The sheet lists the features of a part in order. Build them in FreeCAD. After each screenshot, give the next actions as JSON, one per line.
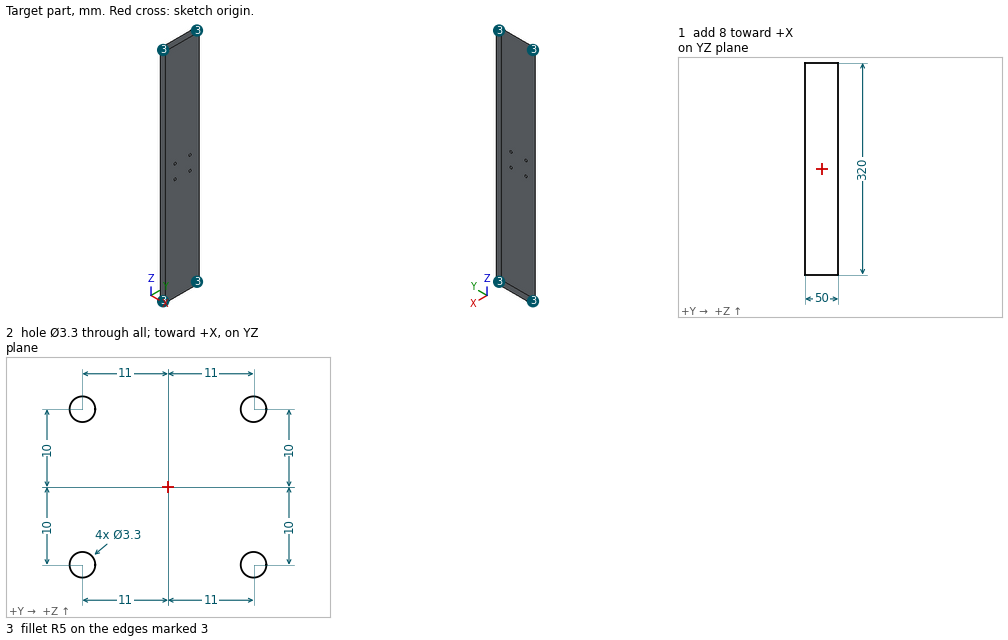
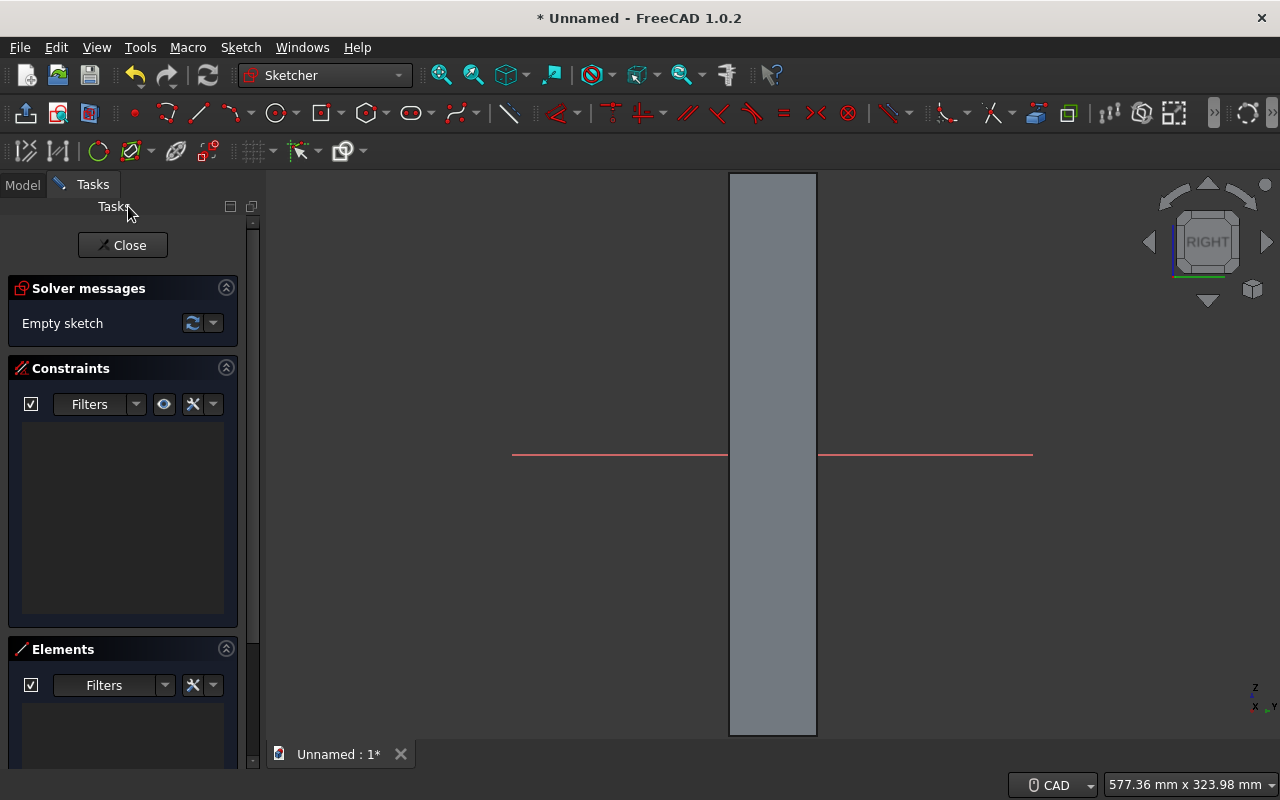
{"action": "left_click", "coordinate": [90, 114]}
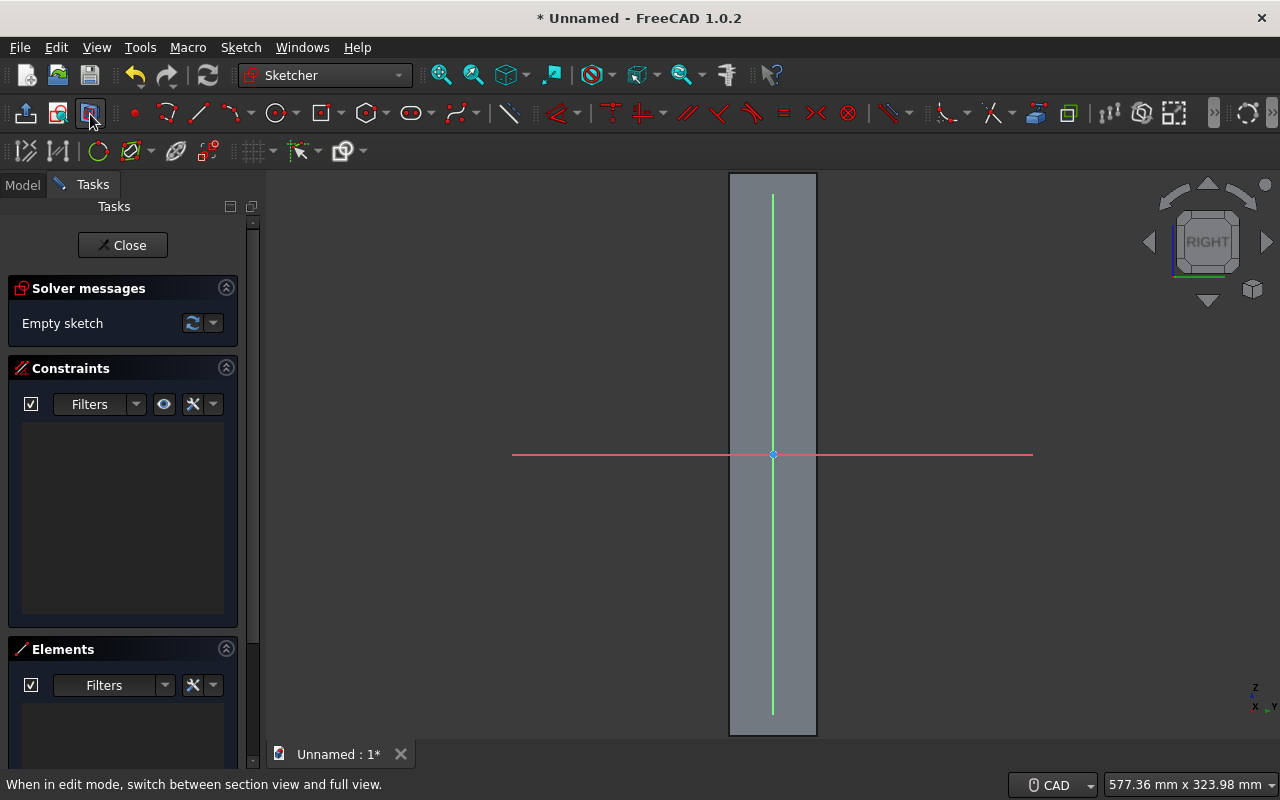
{"action": "scroll", "coordinate": [782, 454], "scroll_direction": "up", "scroll_amount": 11}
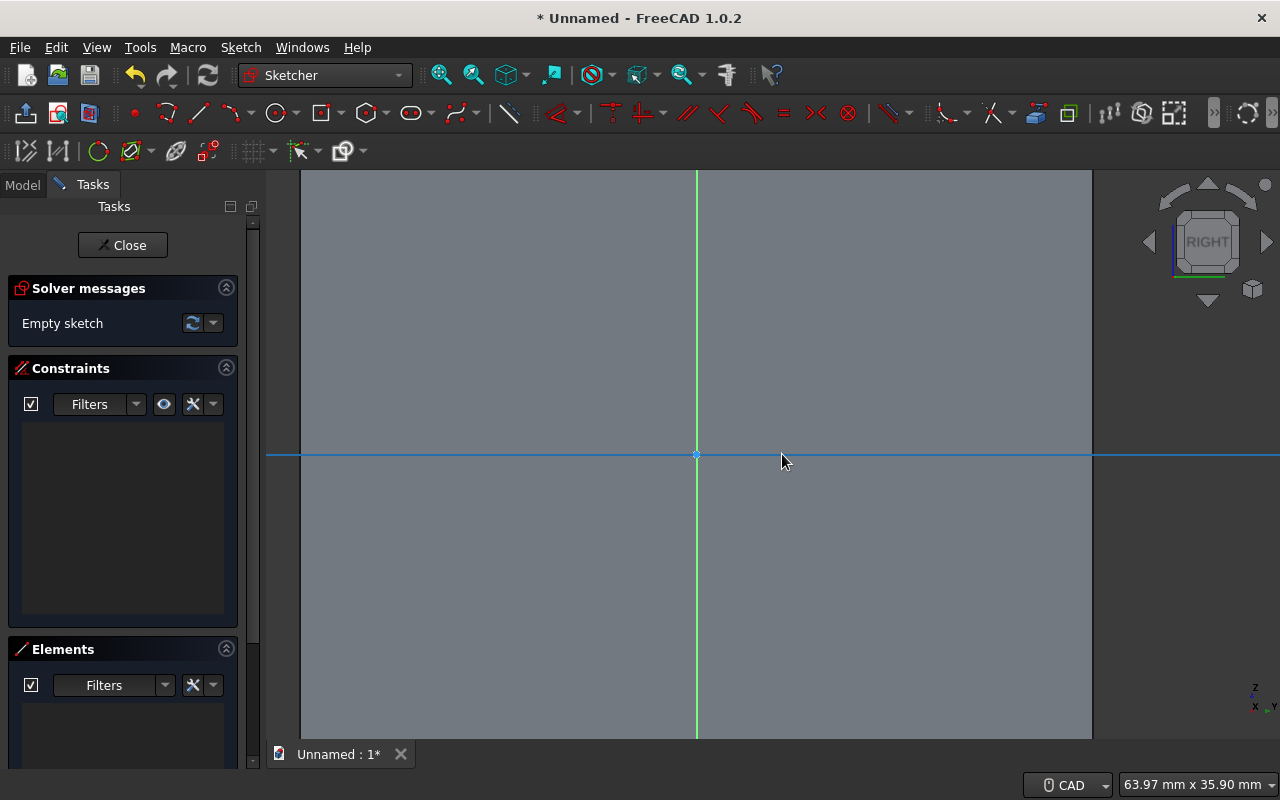
{"action": "left_click", "coordinate": [276, 114]}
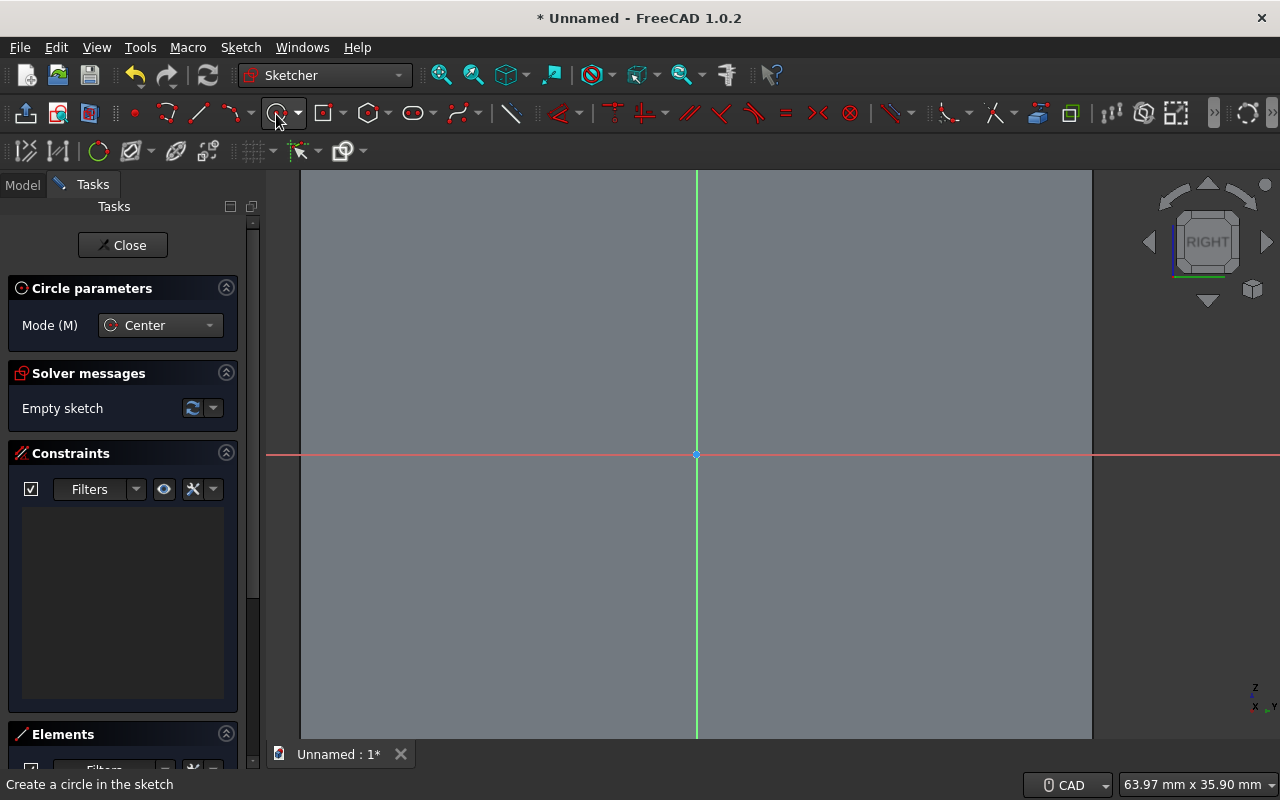
{"action": "left_click", "coordinate": [522, 613]}
{"action": "left_click", "coordinate": [541, 595]}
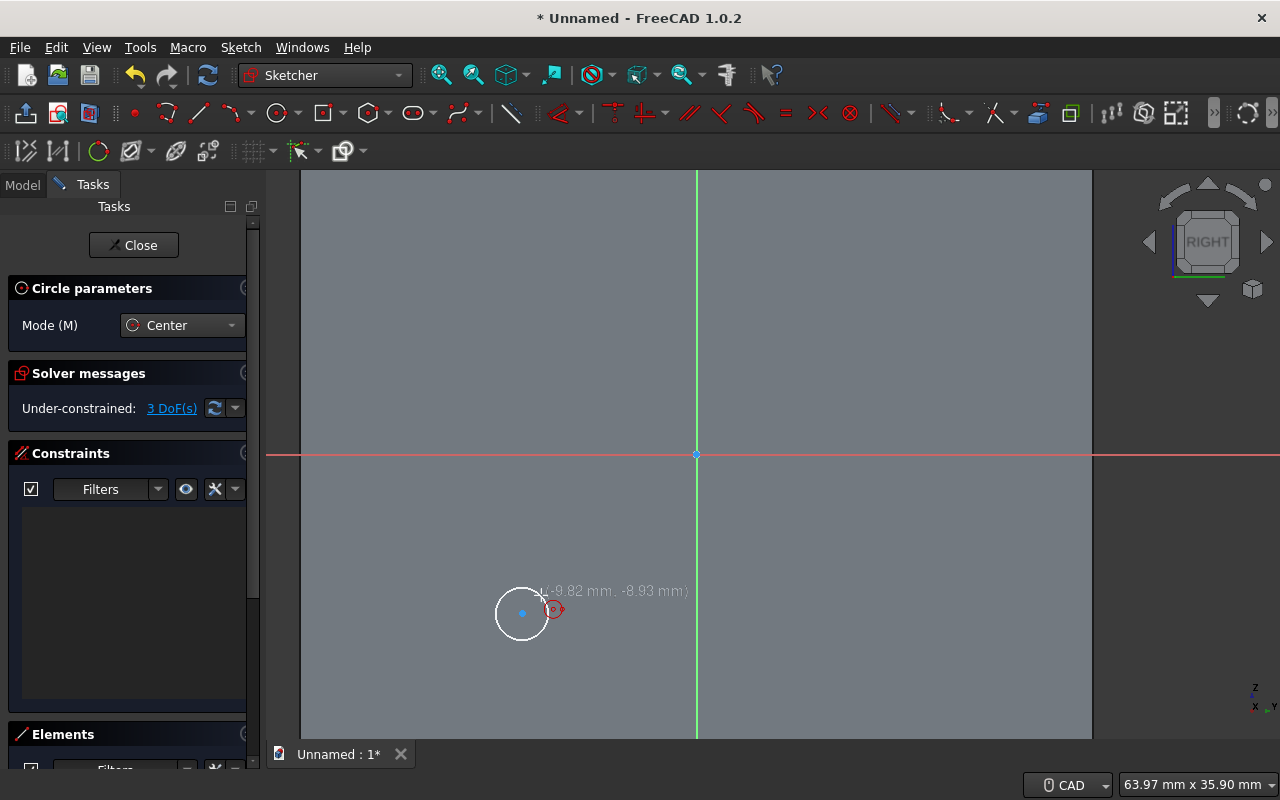
{"action": "left_click", "coordinate": [871, 613]}
{"action": "left_click", "coordinate": [890, 595]}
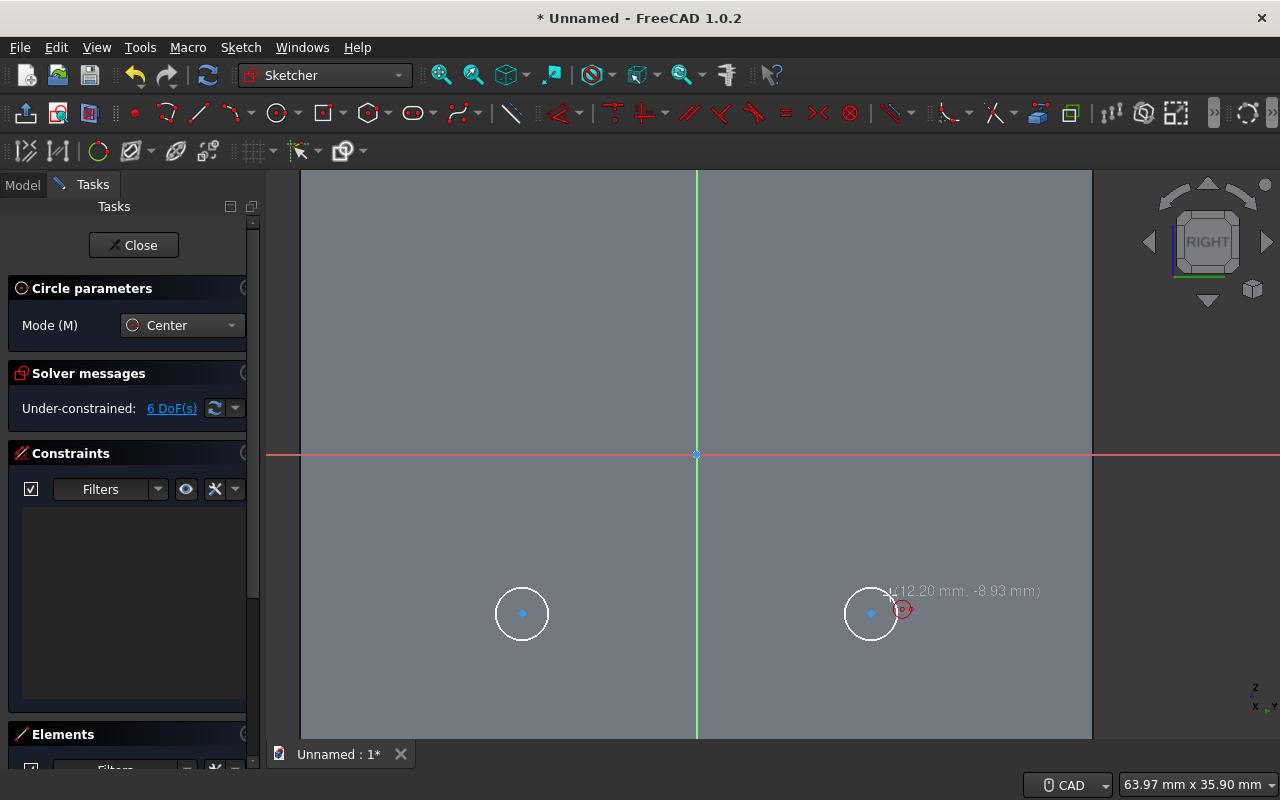
{"action": "left_click", "coordinate": [522, 296]}
{"action": "left_click", "coordinate": [541, 278]}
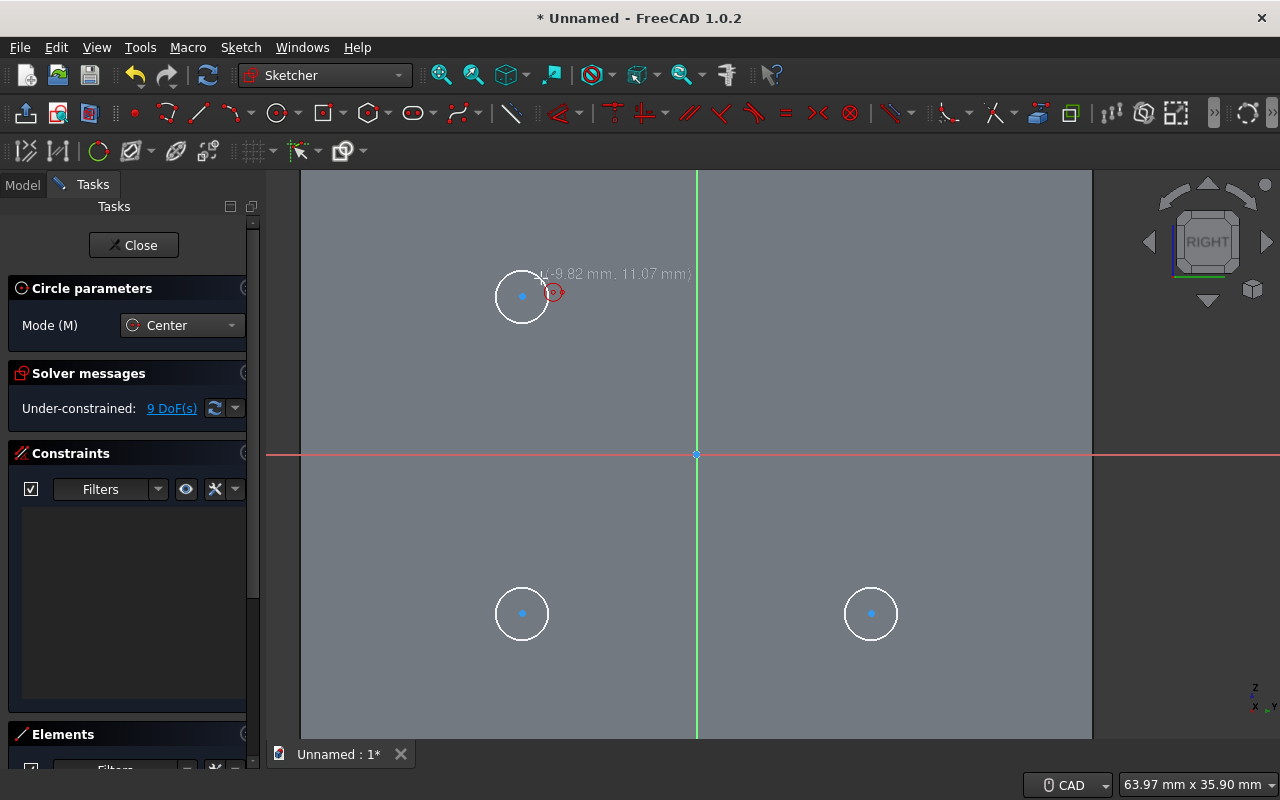
{"action": "left_click", "coordinate": [871, 296]}
{"action": "left_click", "coordinate": [890, 278]}
{"action": "key", "text": "Escape"}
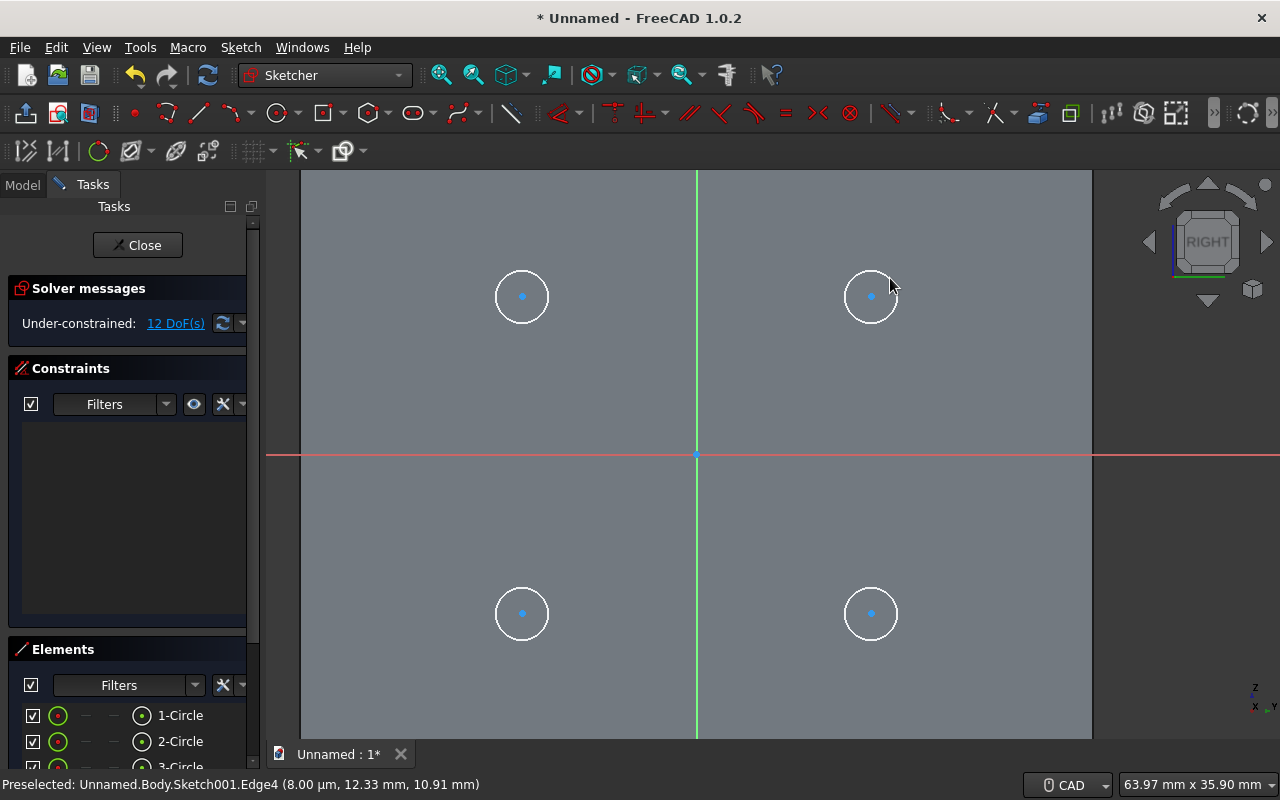
{"action": "left_click", "coordinate": [540, 595]}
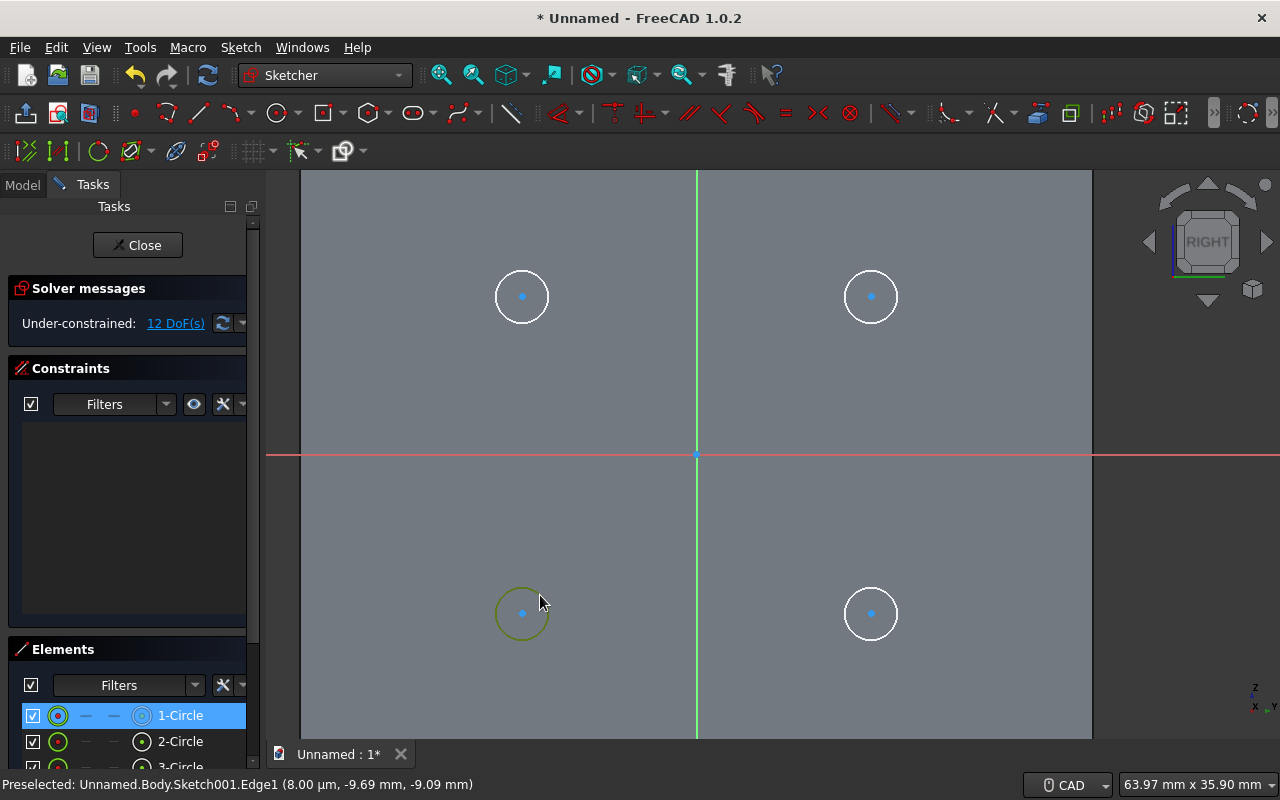
{"action": "left_click", "coordinate": [889, 595]}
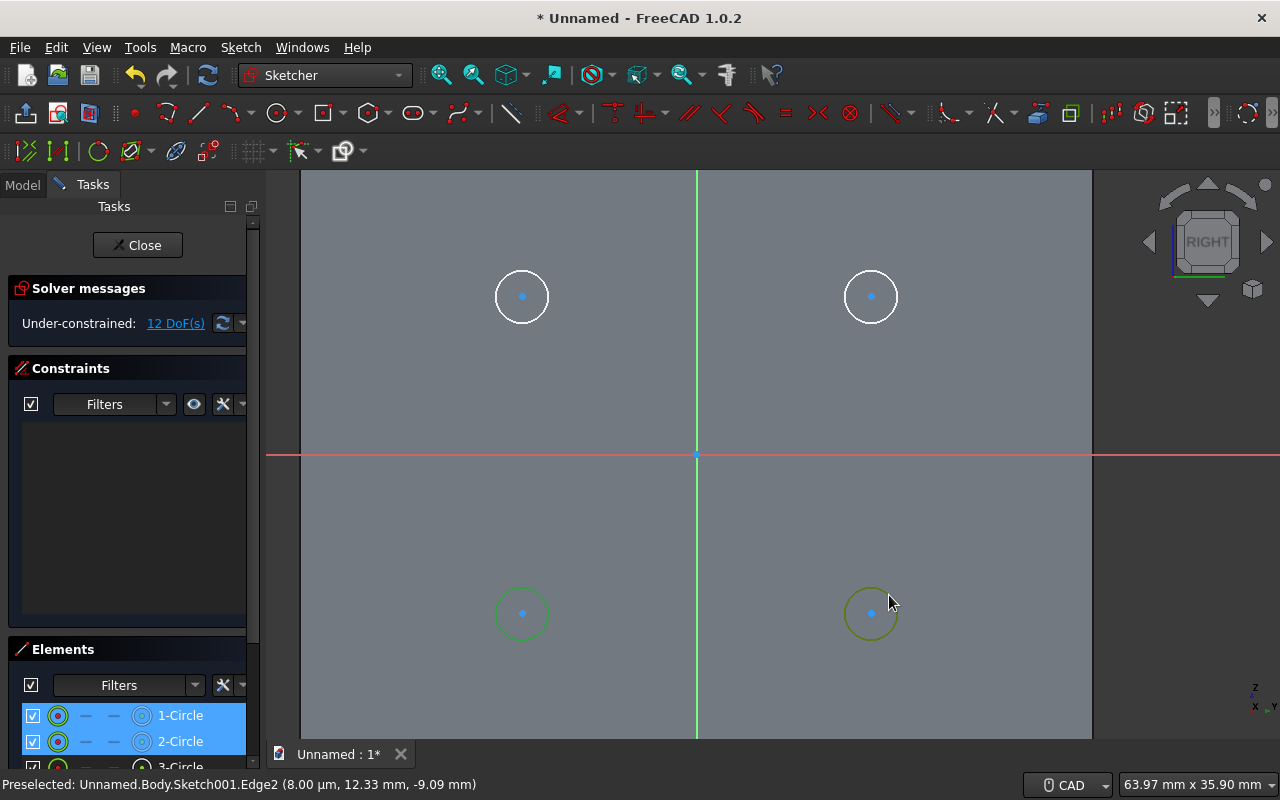
{"action": "left_click", "coordinate": [540, 278]}